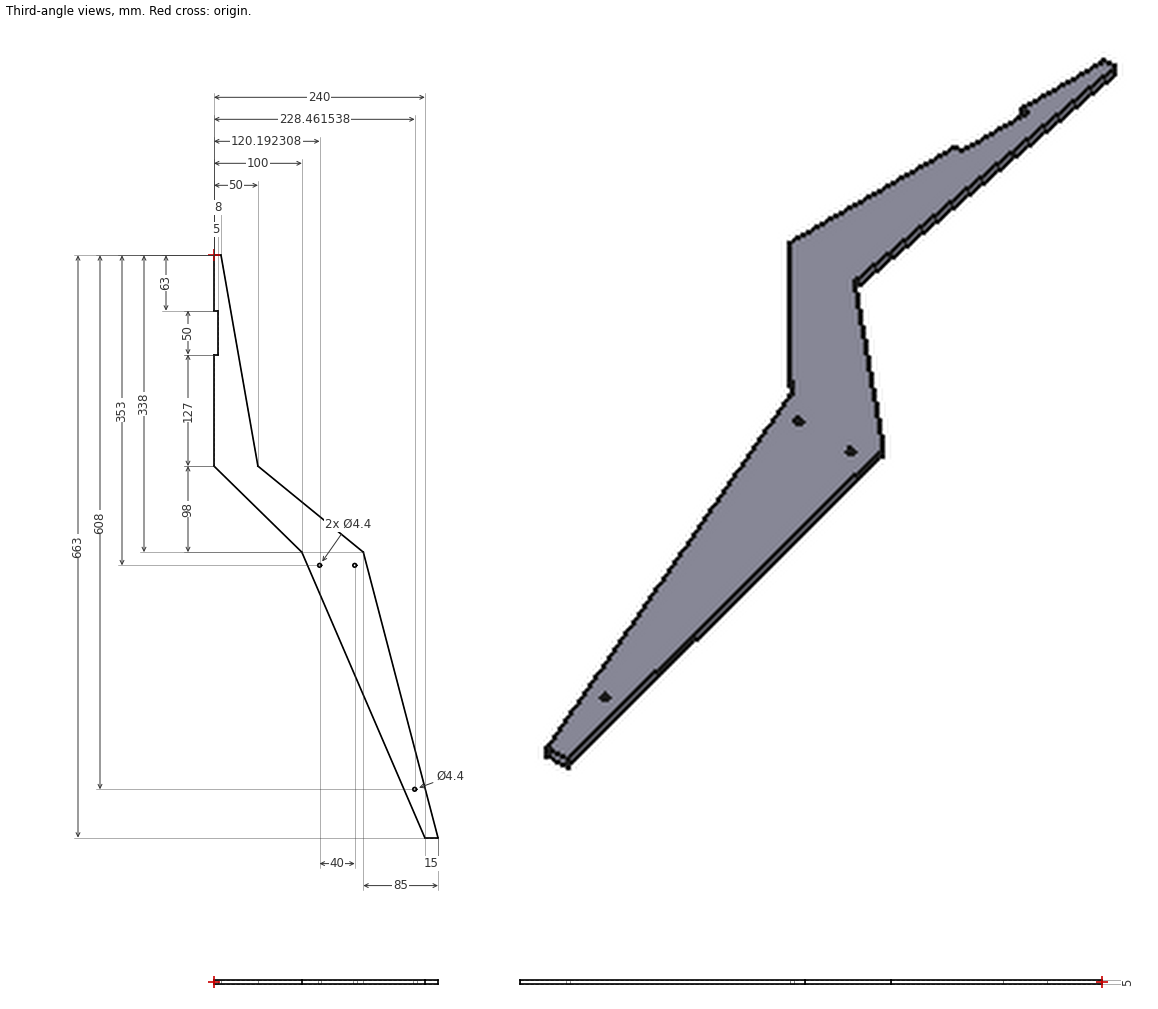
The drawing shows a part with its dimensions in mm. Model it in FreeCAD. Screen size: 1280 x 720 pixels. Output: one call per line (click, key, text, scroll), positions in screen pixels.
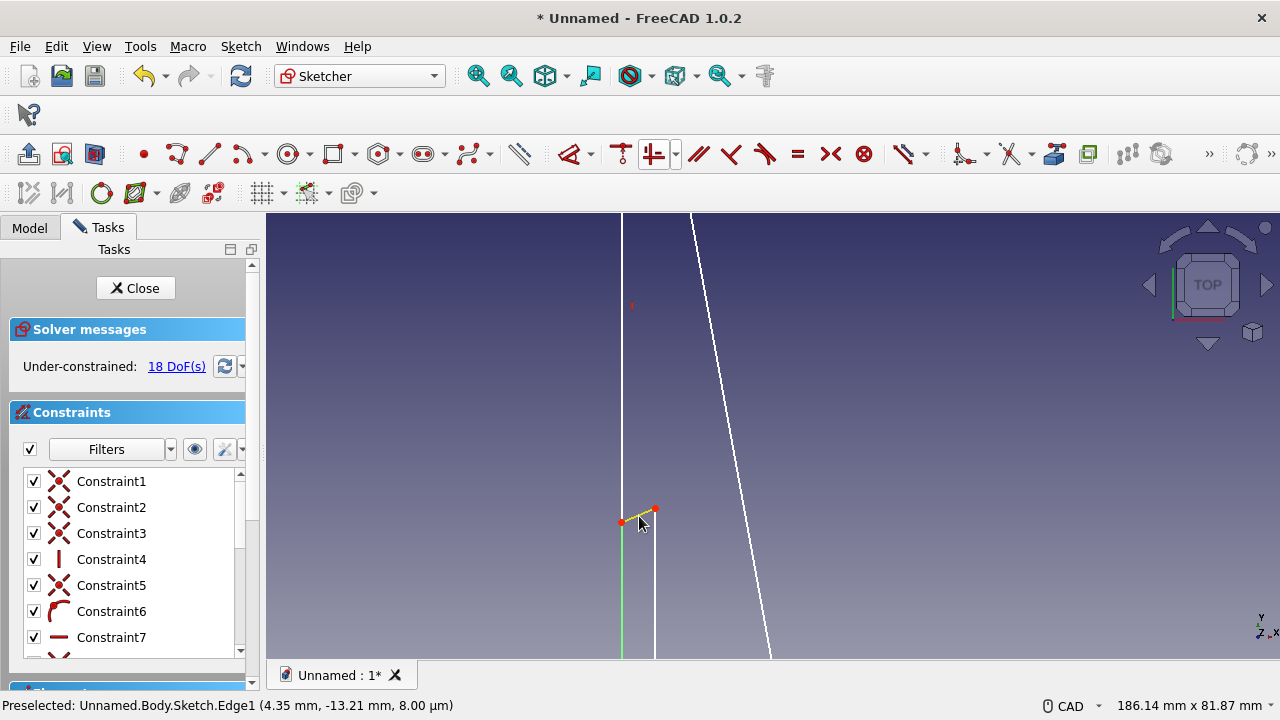
click(638, 516)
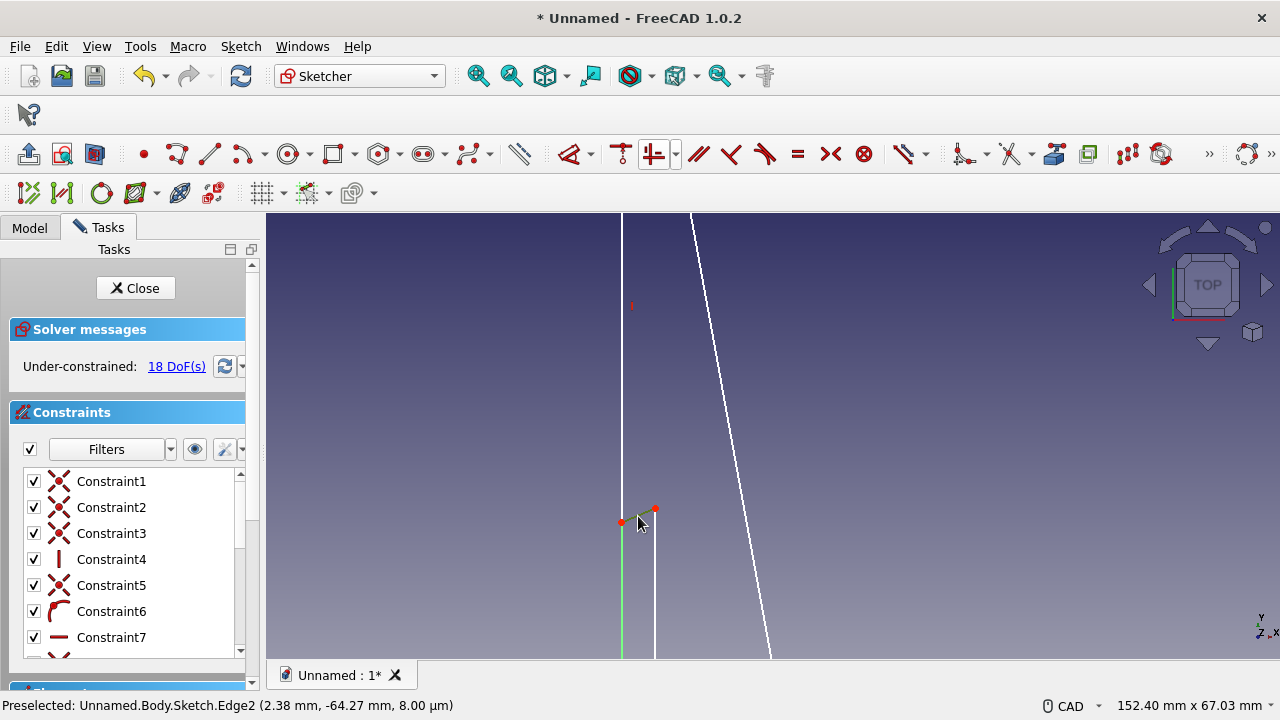
click(676, 154)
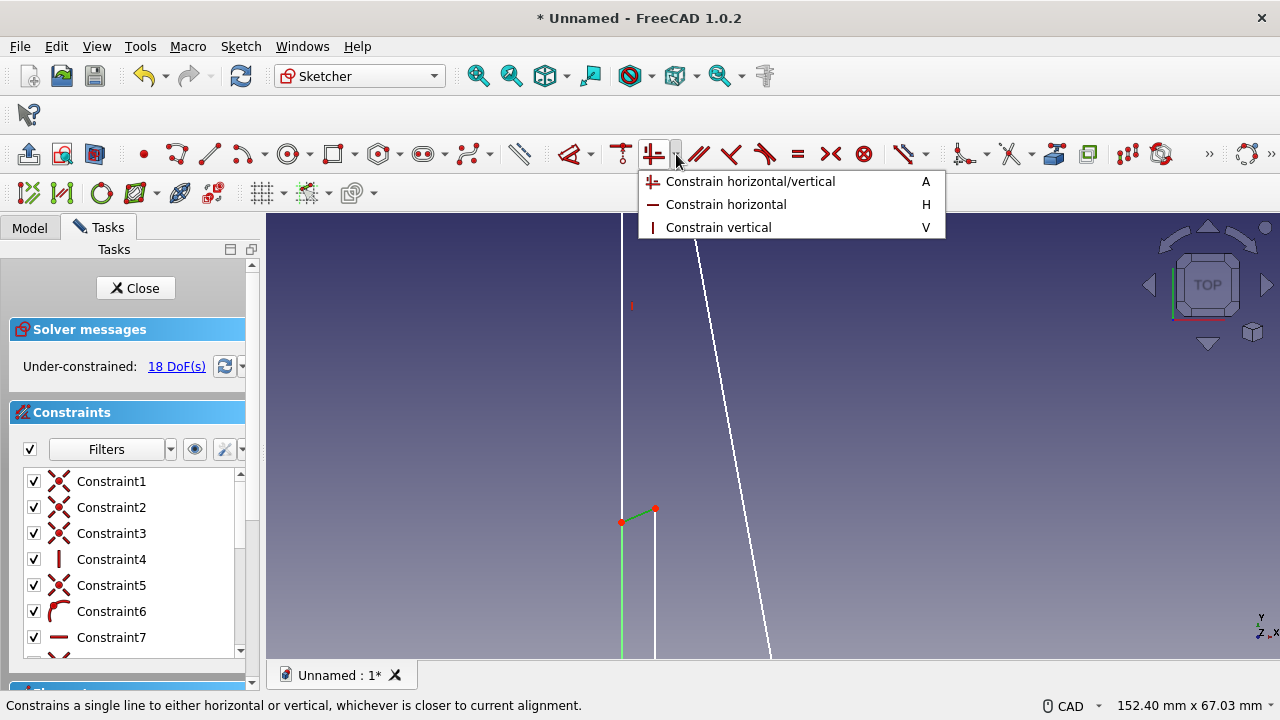
click(792, 204)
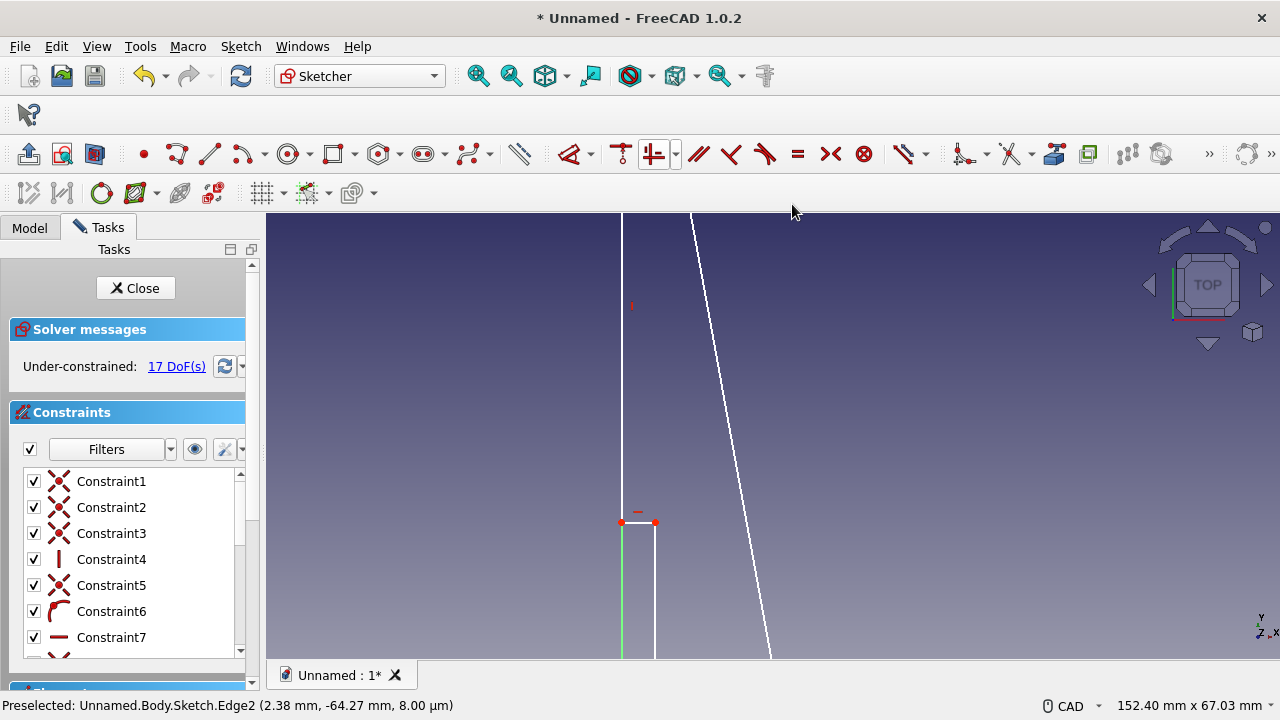
scroll(655, 316, down, 14)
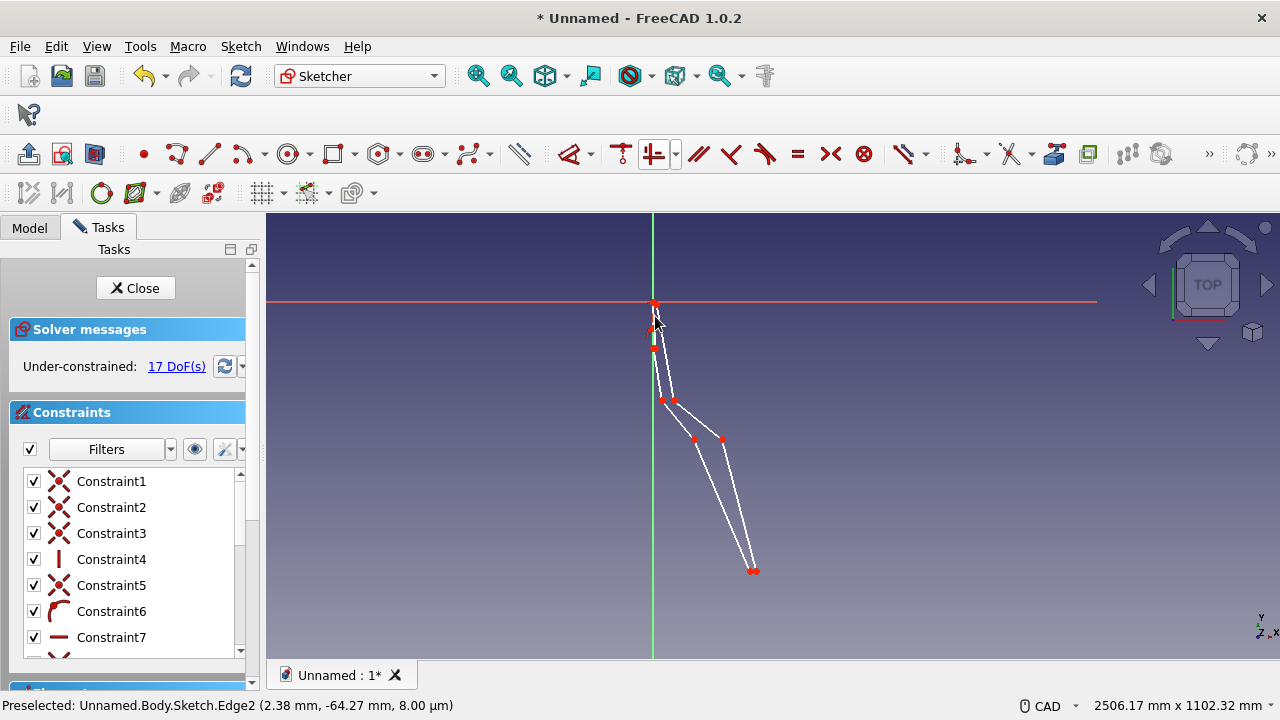
scroll(656, 364, up, 9)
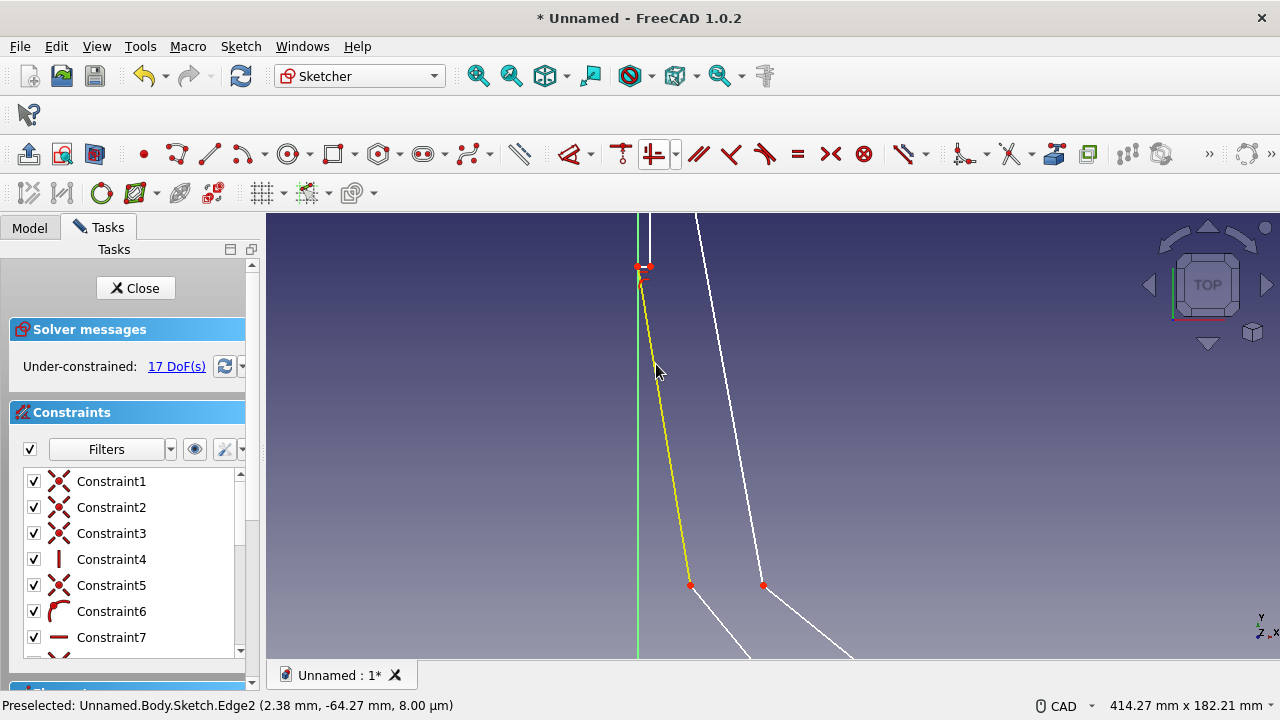
click(654, 362)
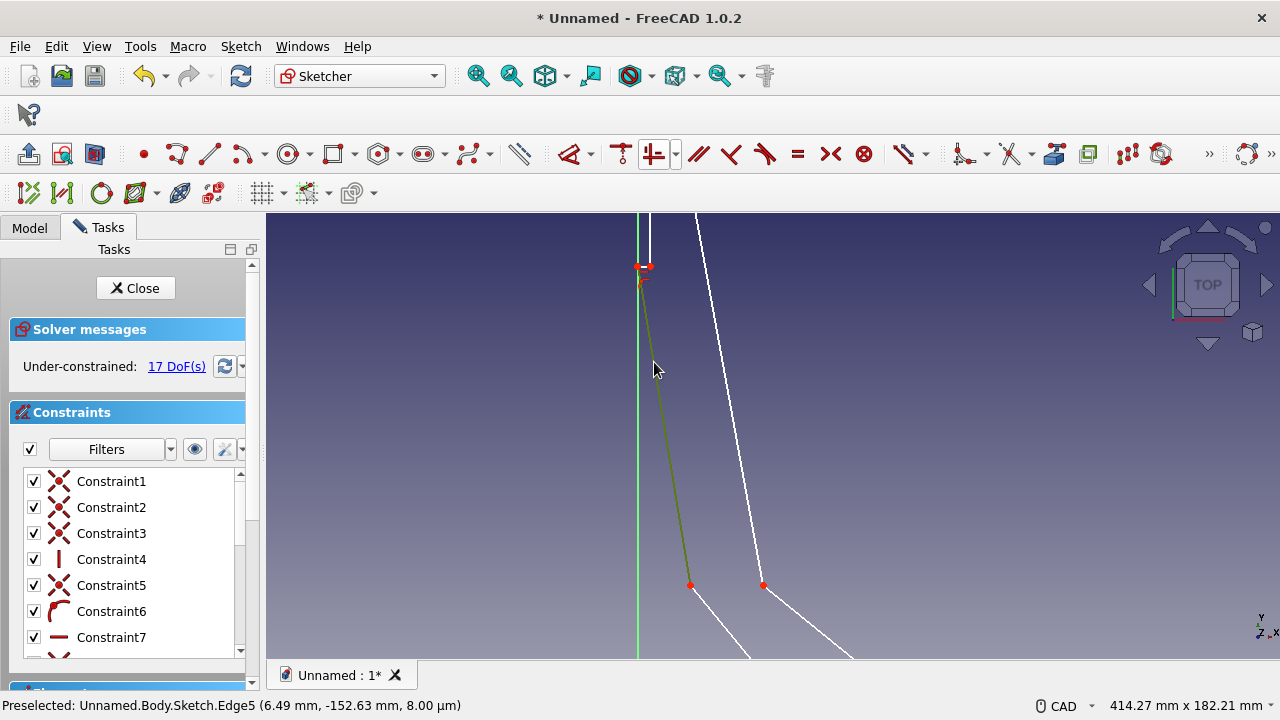
click(676, 154)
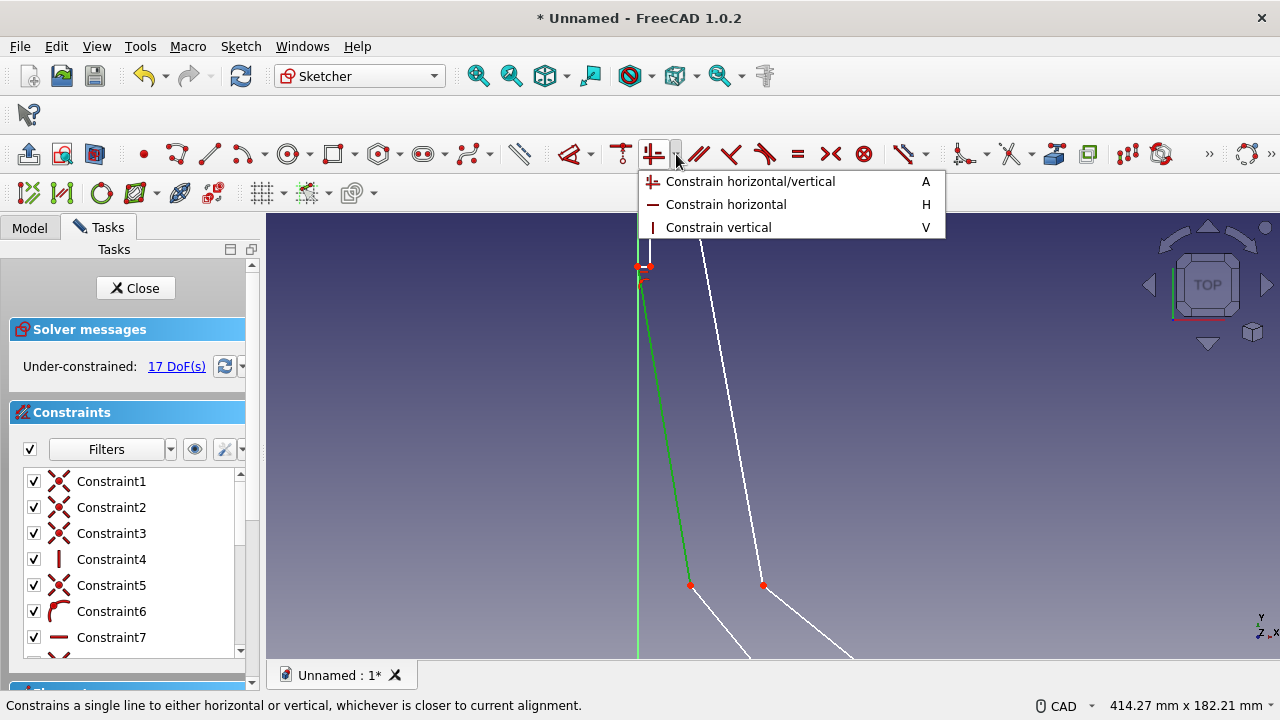
click(792, 228)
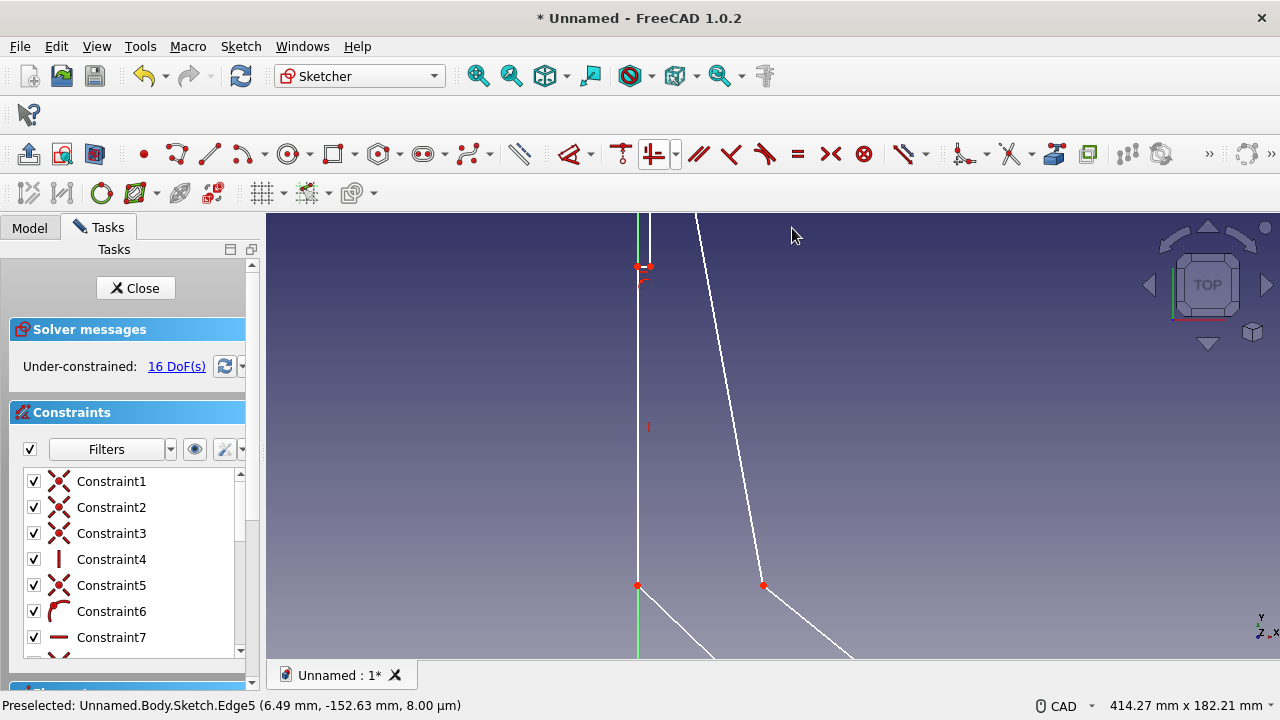
scroll(656, 364, down, 9)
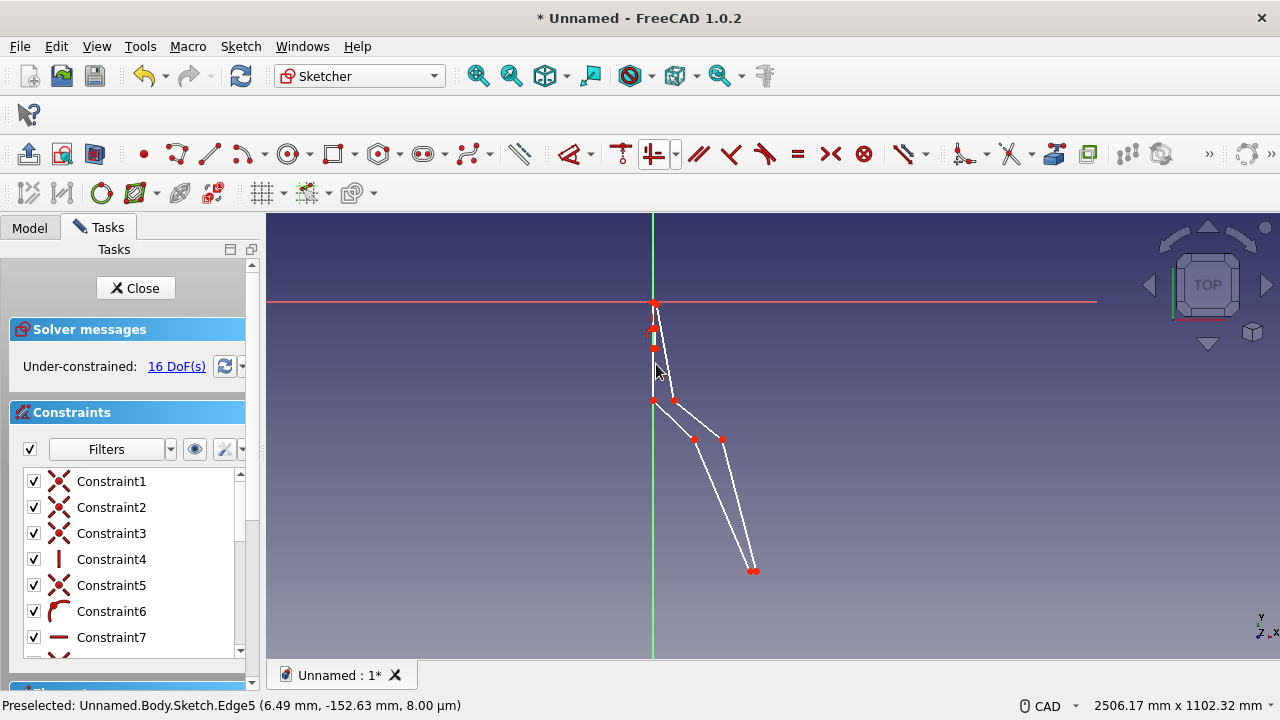
scroll(752, 572, up, 10)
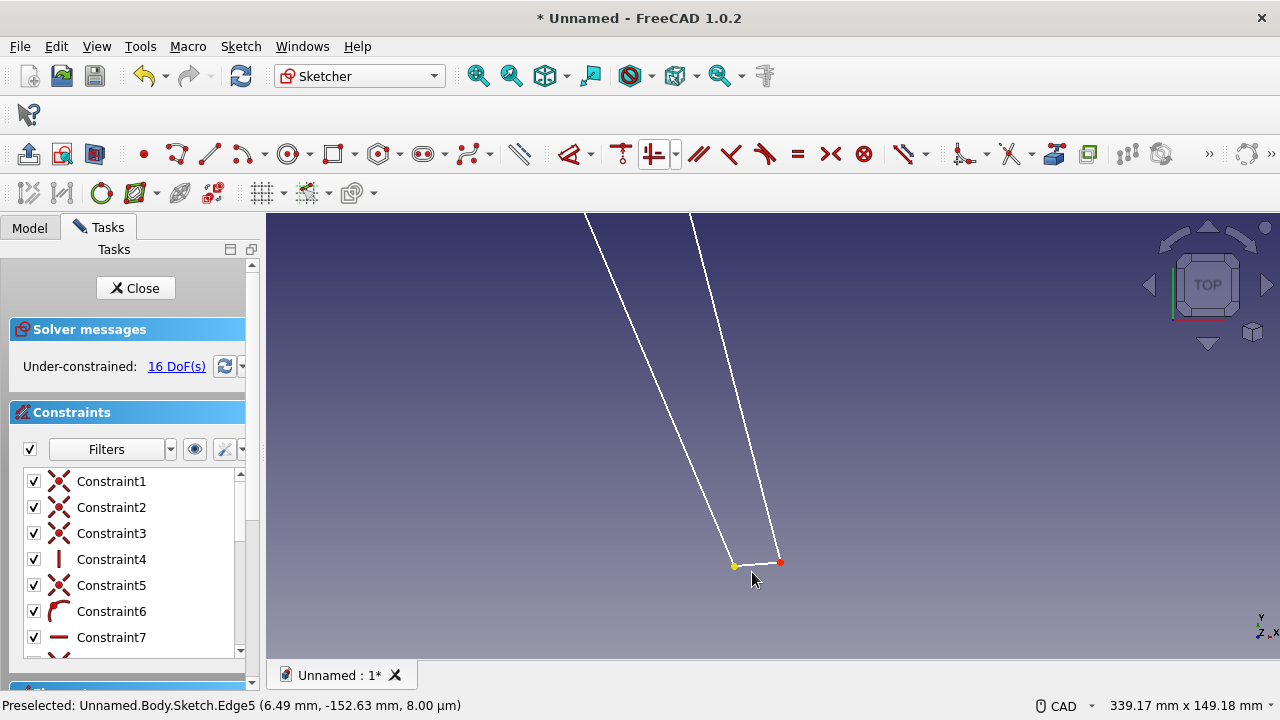
click(748, 565)